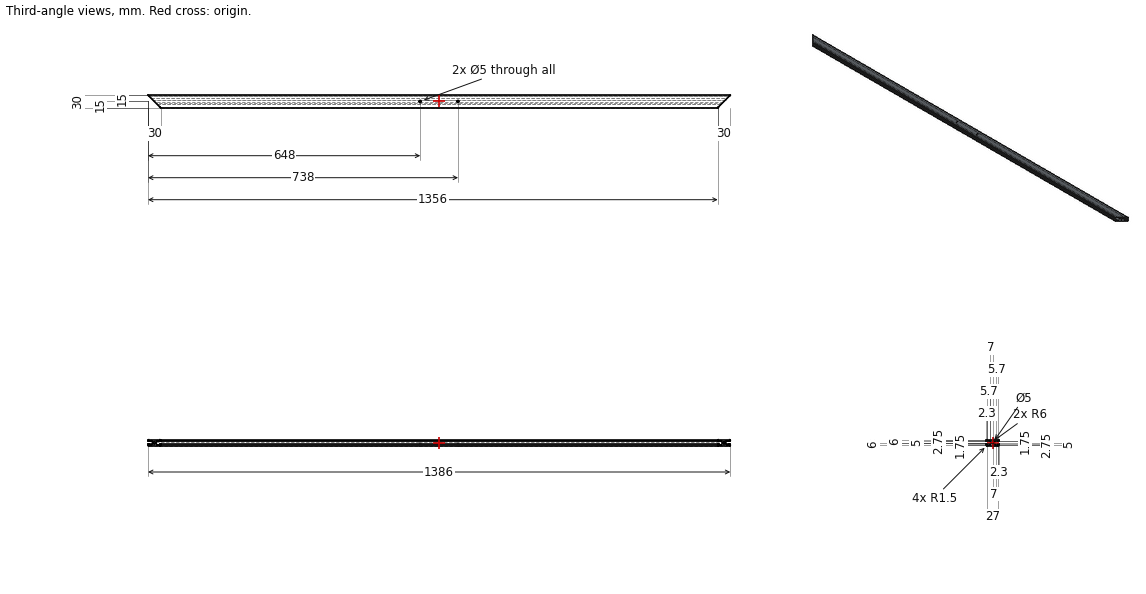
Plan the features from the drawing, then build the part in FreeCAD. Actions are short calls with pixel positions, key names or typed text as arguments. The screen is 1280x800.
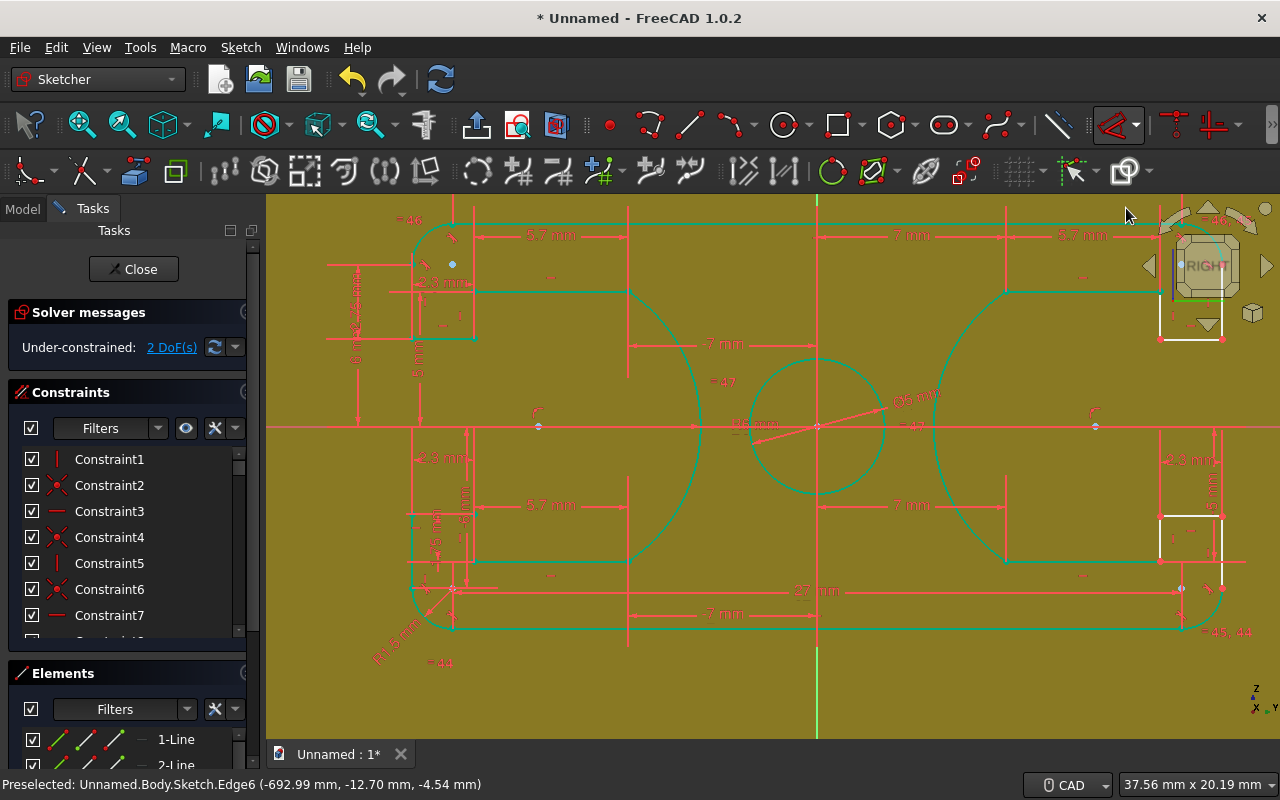
scroll(475, 548, down, 2)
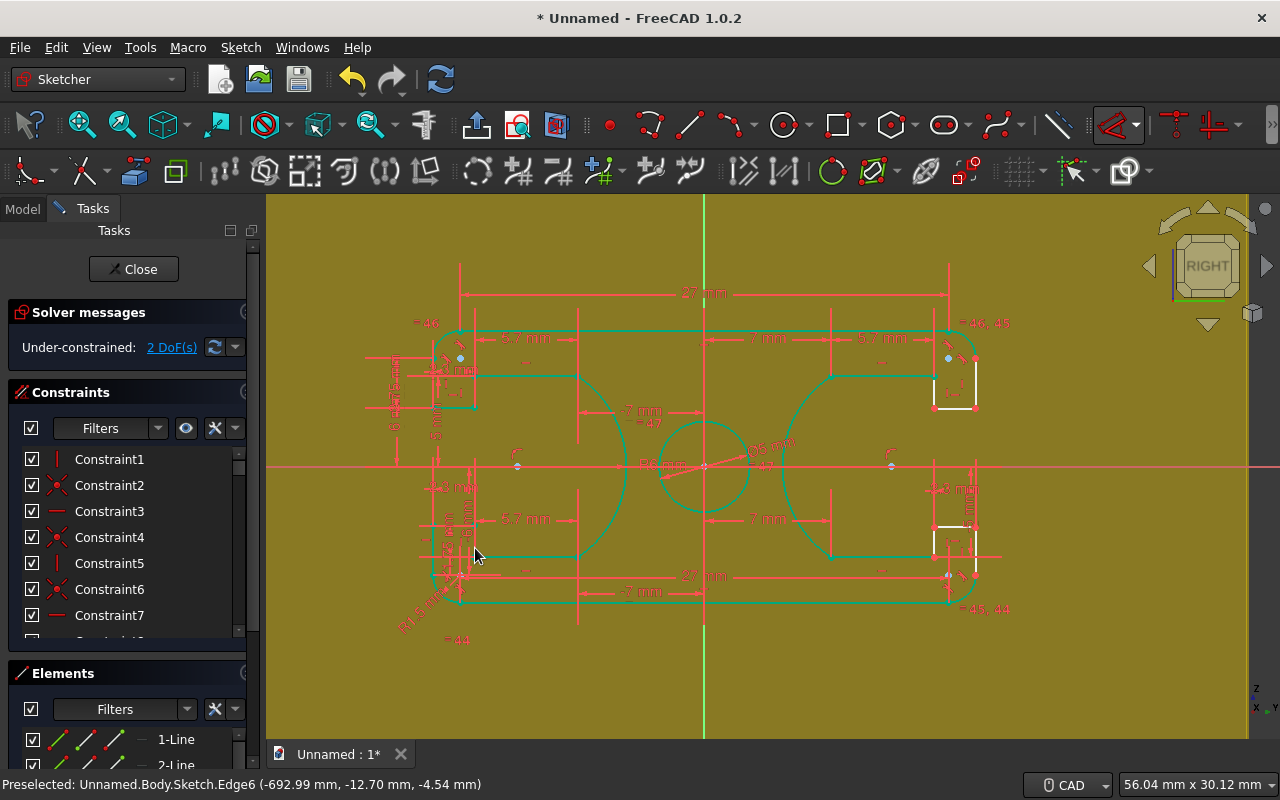
click(976, 561)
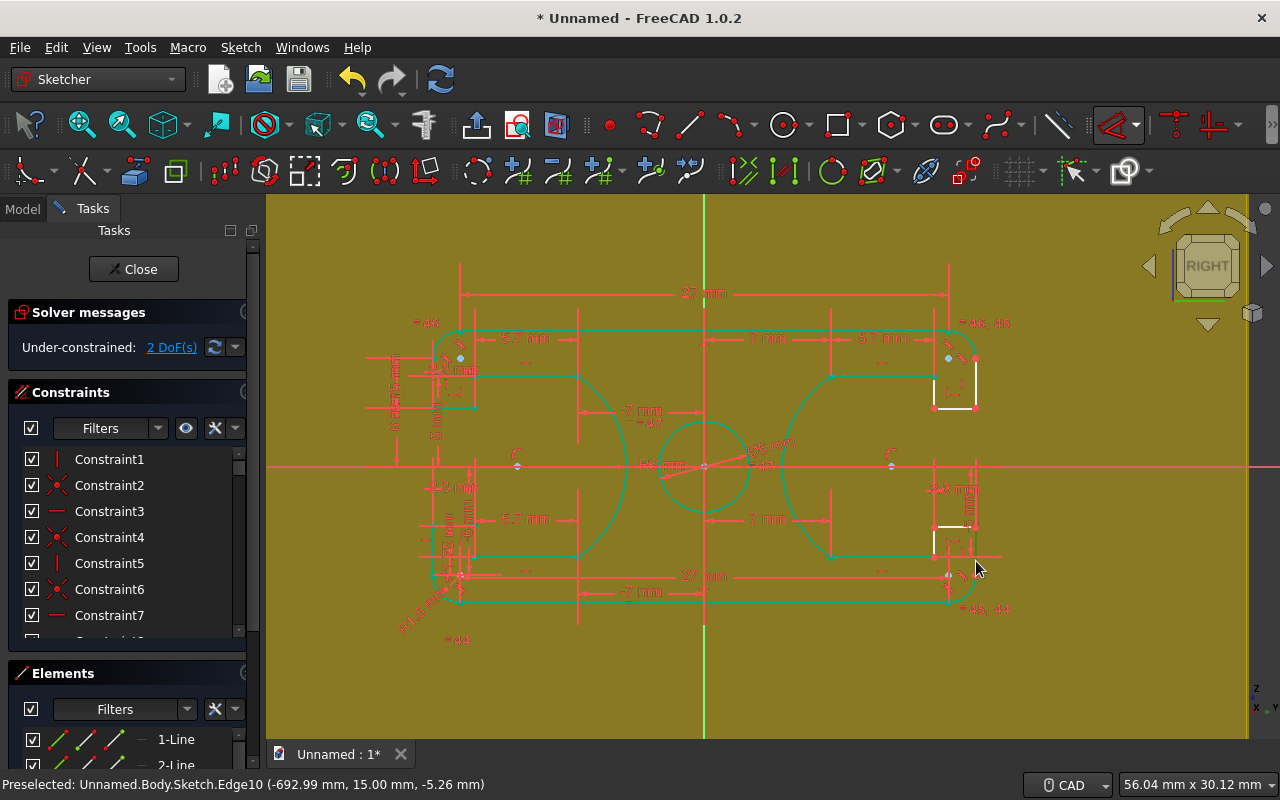
key(i)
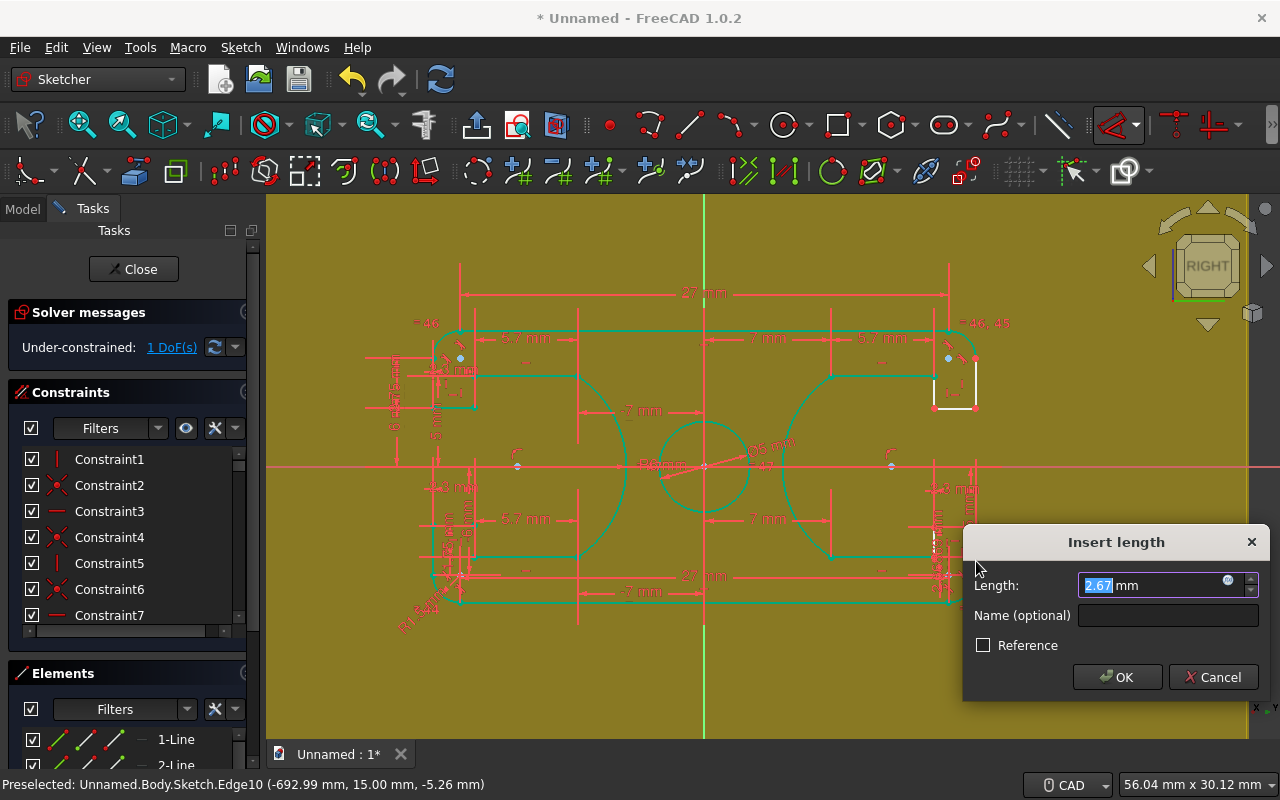
text(2.75)
key(Return)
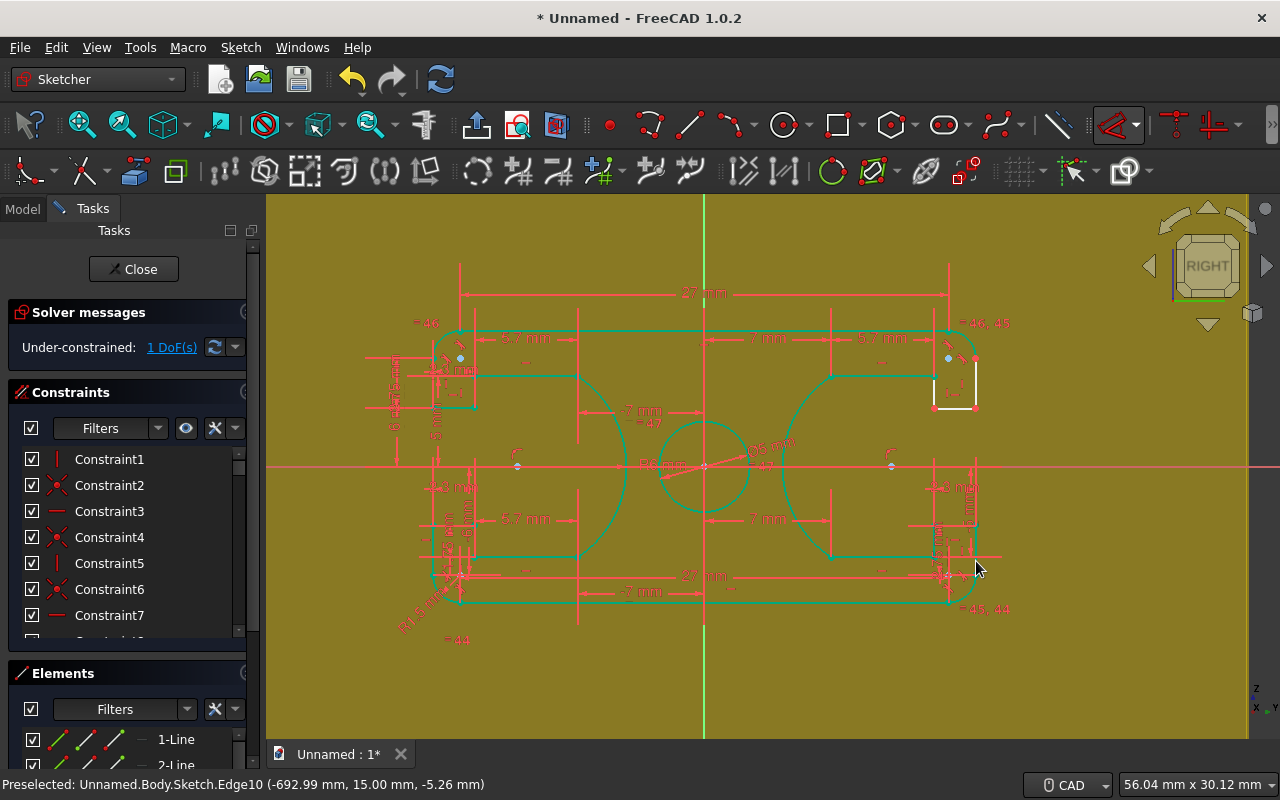
scroll(934, 386, up, 2)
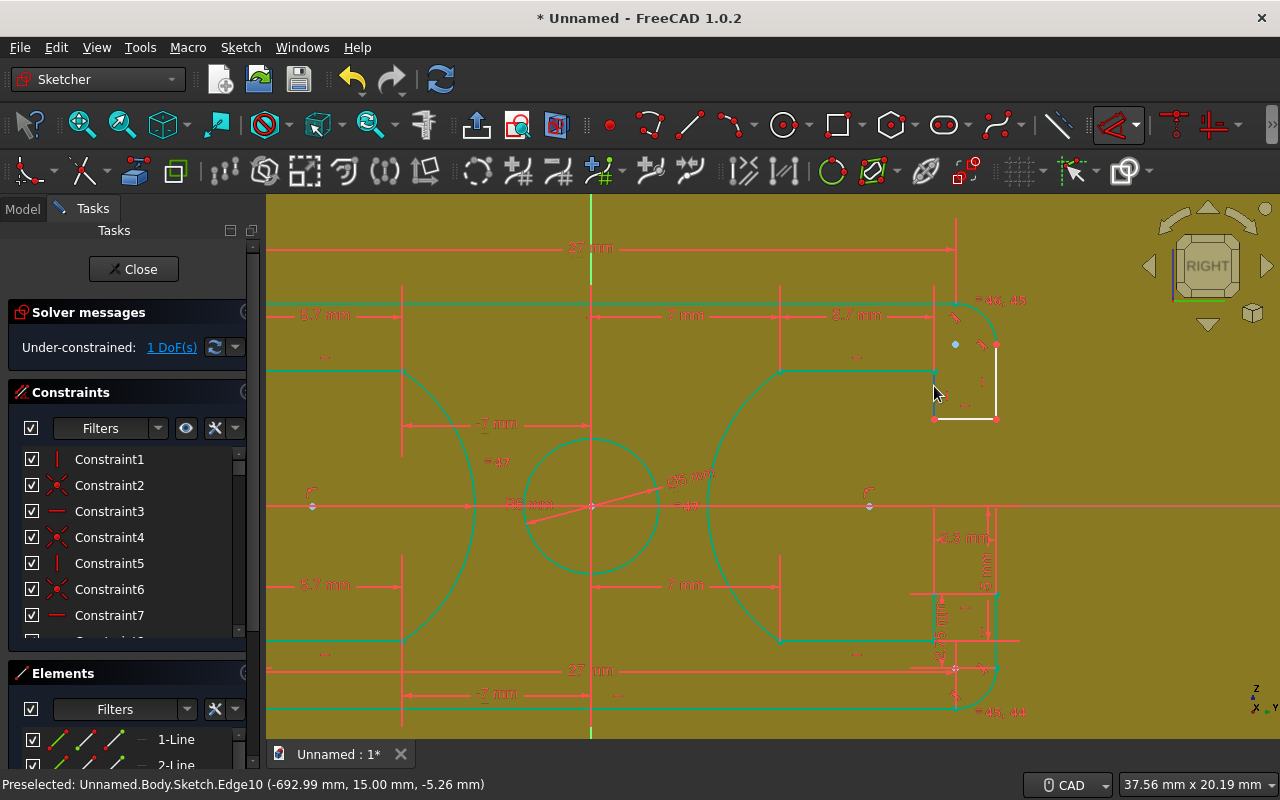
click(934, 386)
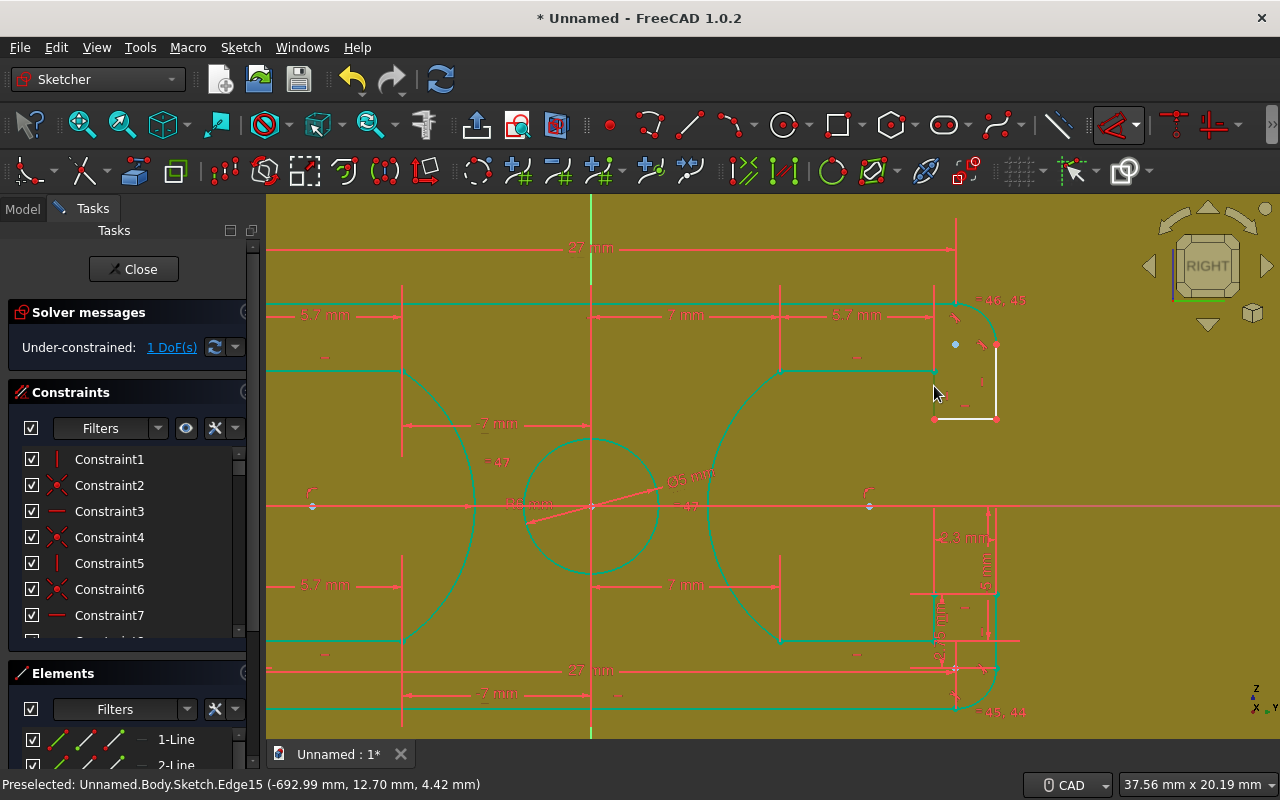
key(i)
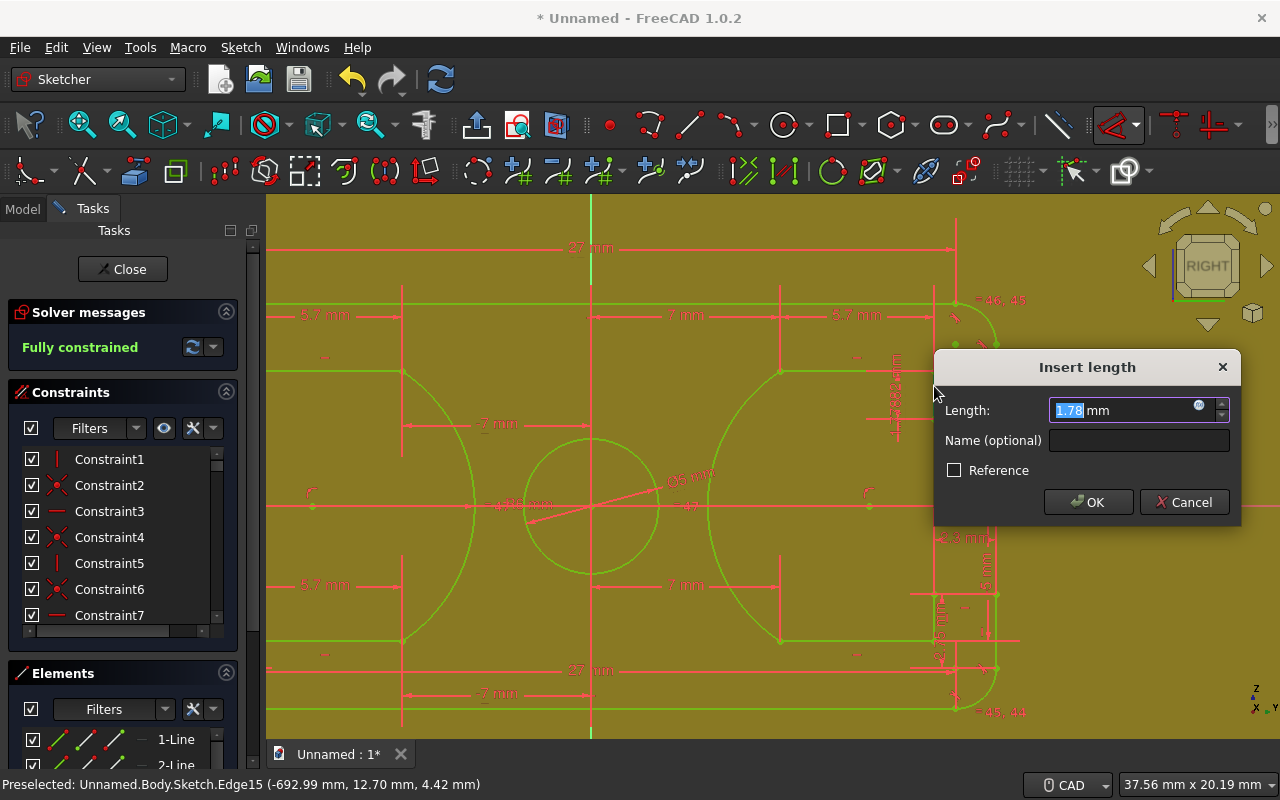
text(1.75)
key(Return)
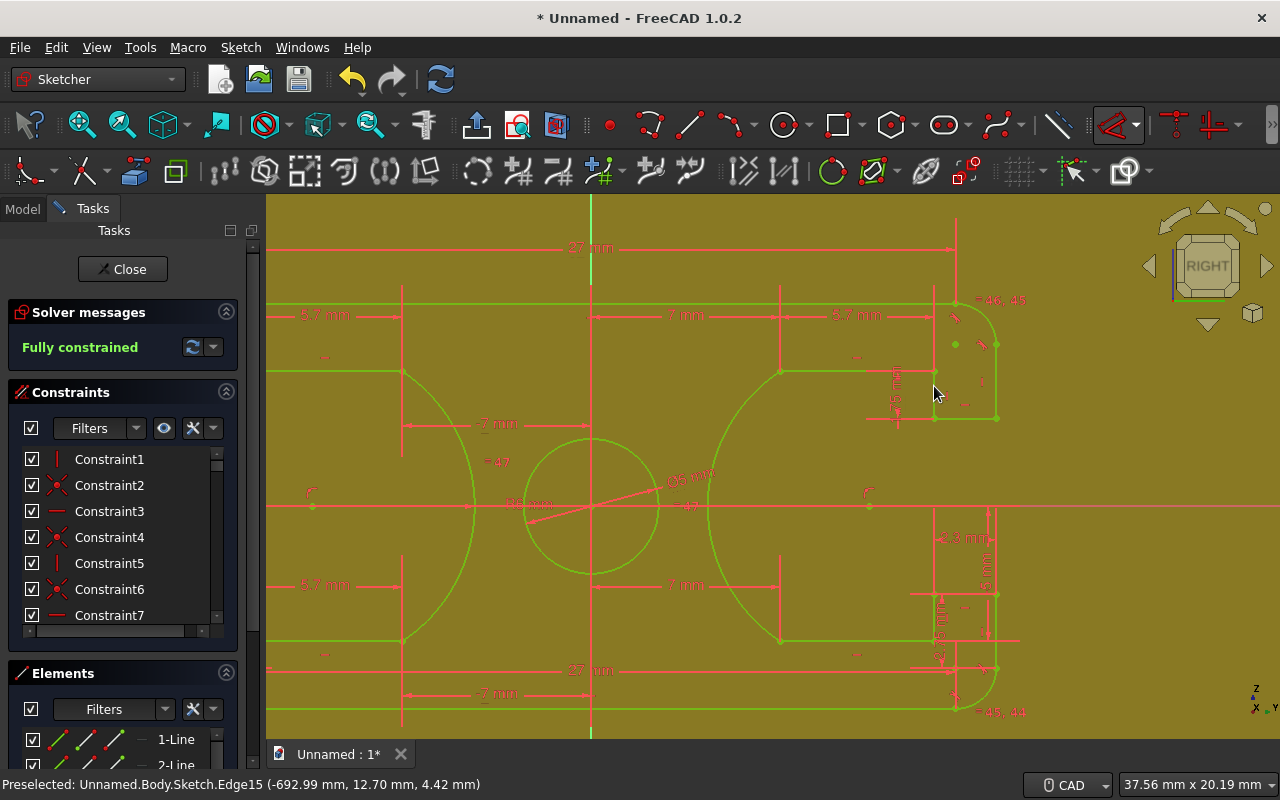
click(123, 269)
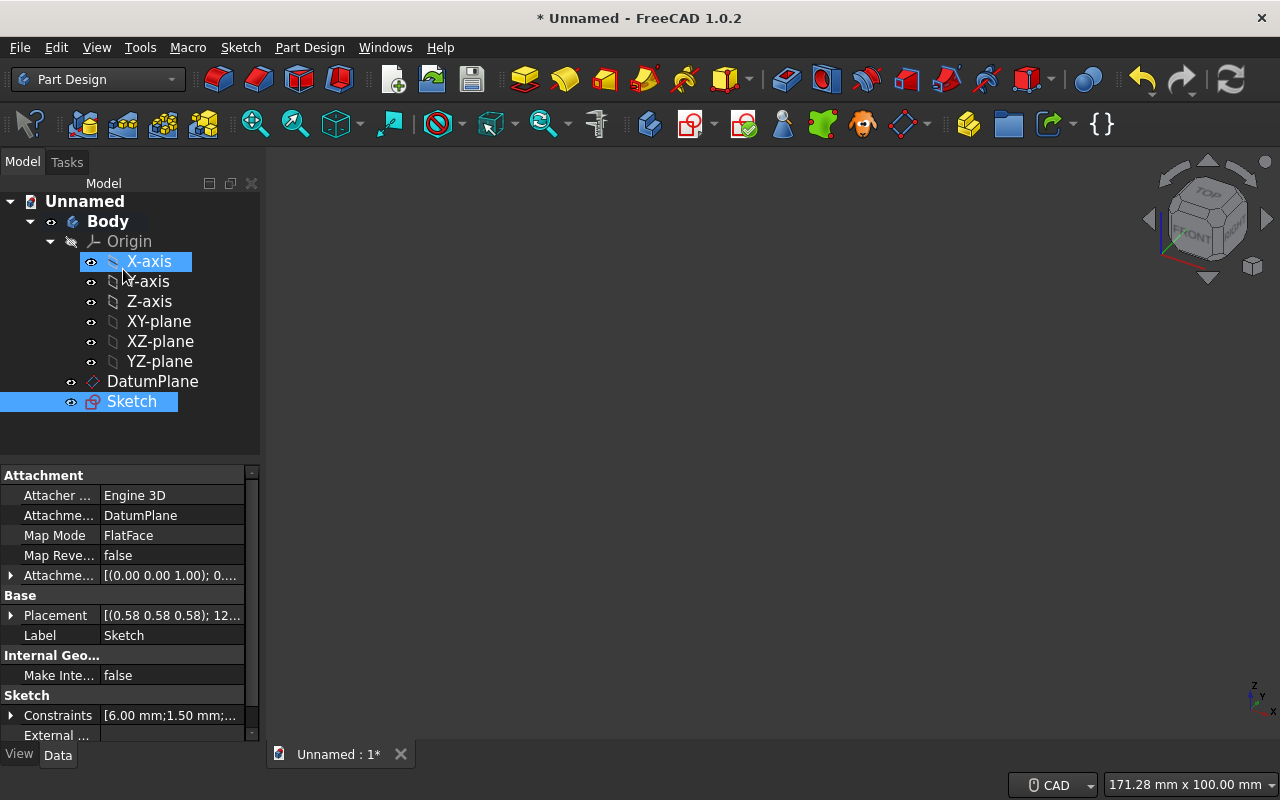
click(526, 80)